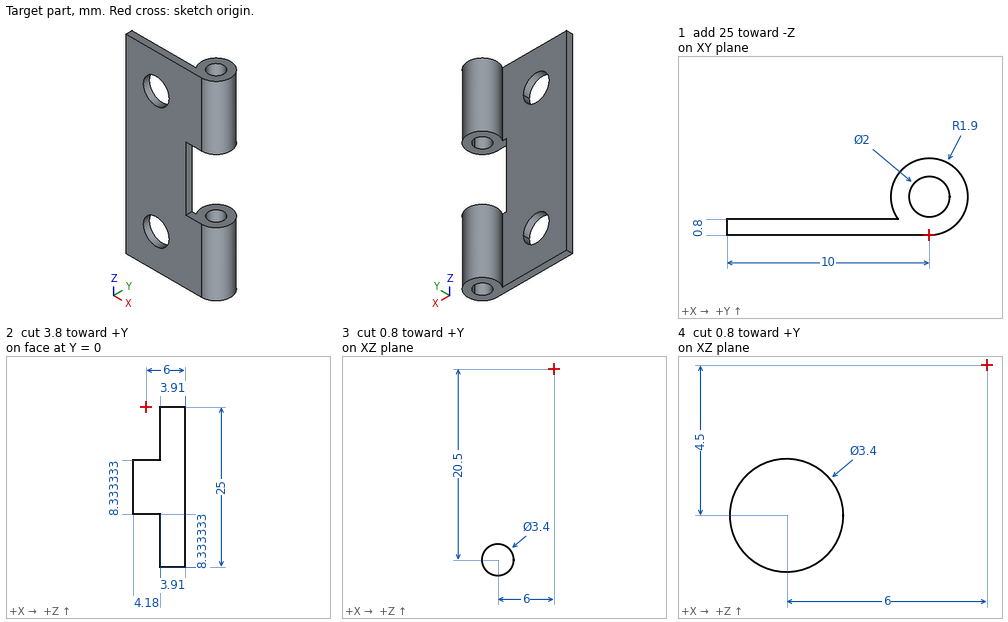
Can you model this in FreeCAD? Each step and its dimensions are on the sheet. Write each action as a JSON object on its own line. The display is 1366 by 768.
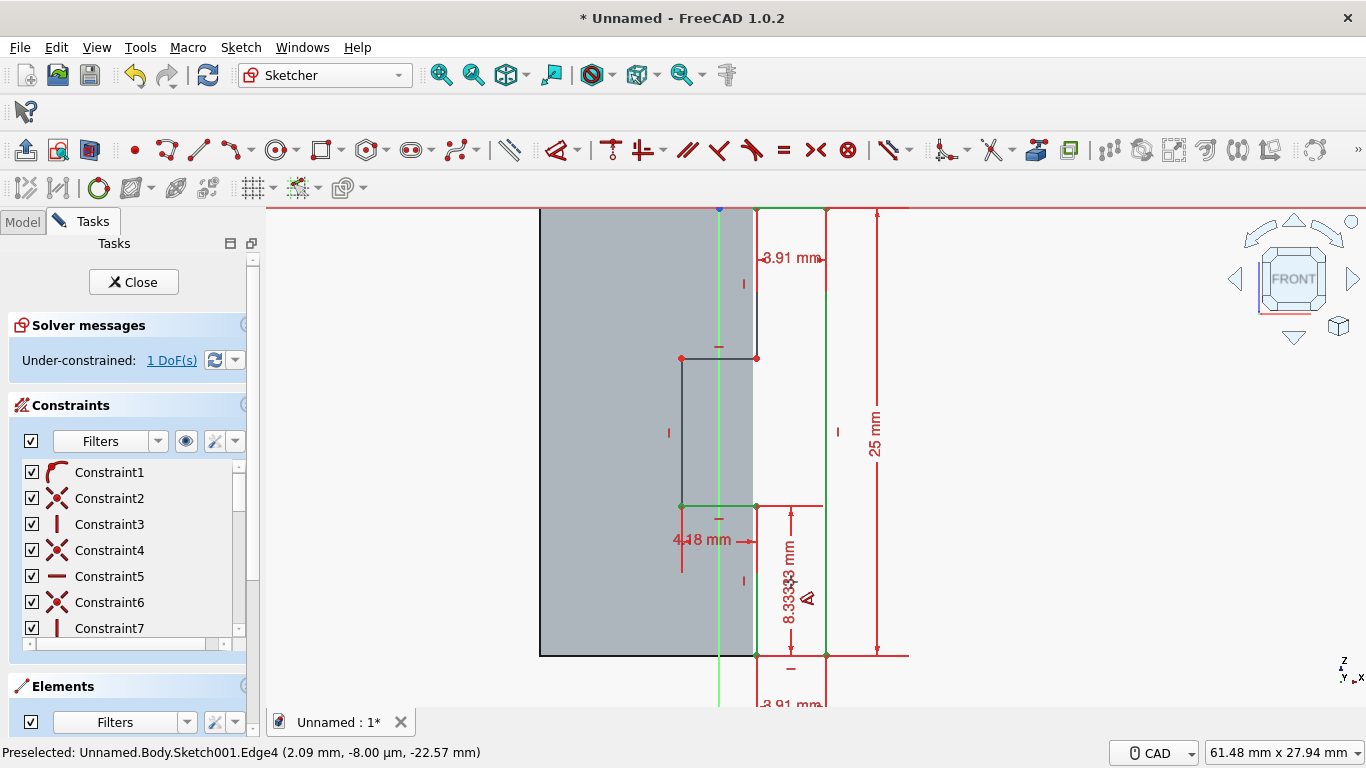
{"action": "left_click", "coordinate": [682, 462]}
{"action": "left_click", "coordinate": [648, 432]}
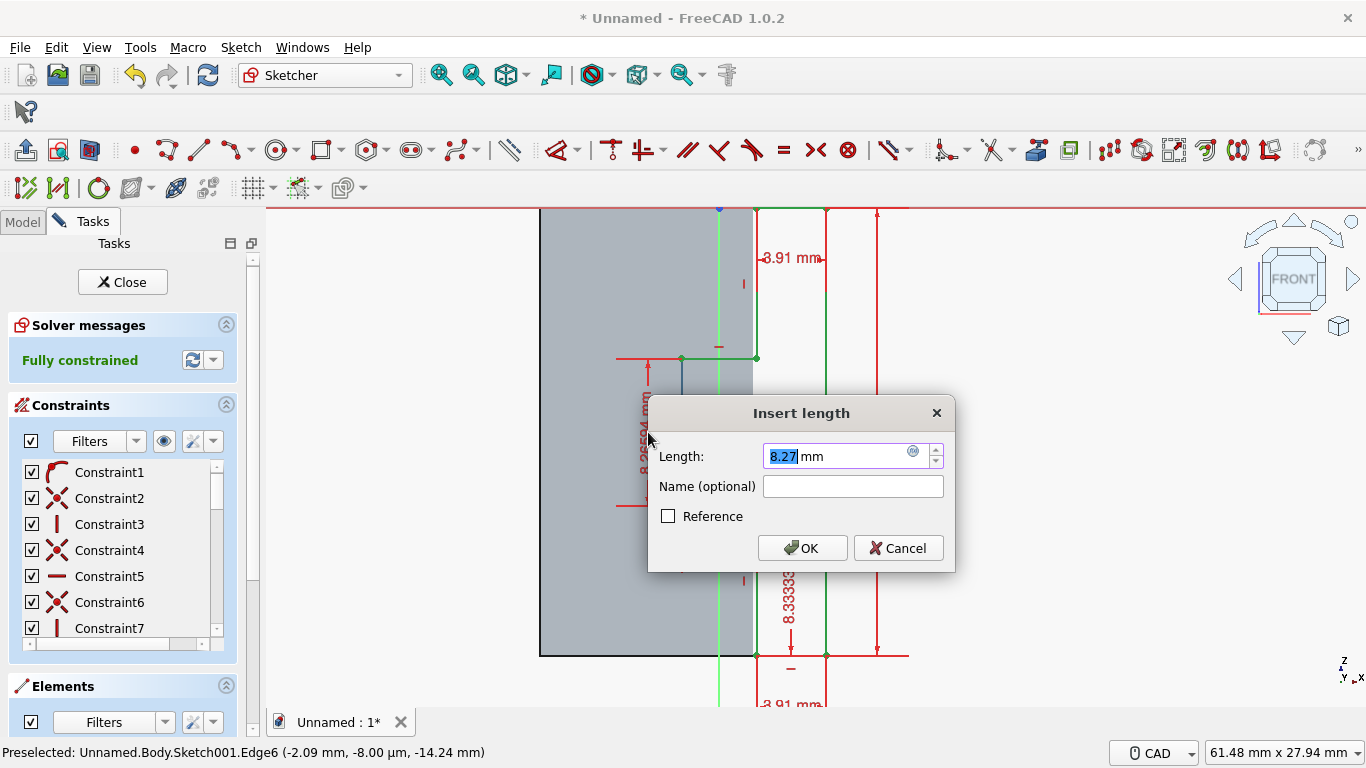
{"action": "type", "text": "8.333333"}
{"action": "key", "text": "Return"}
{"action": "key", "text": "Escape"}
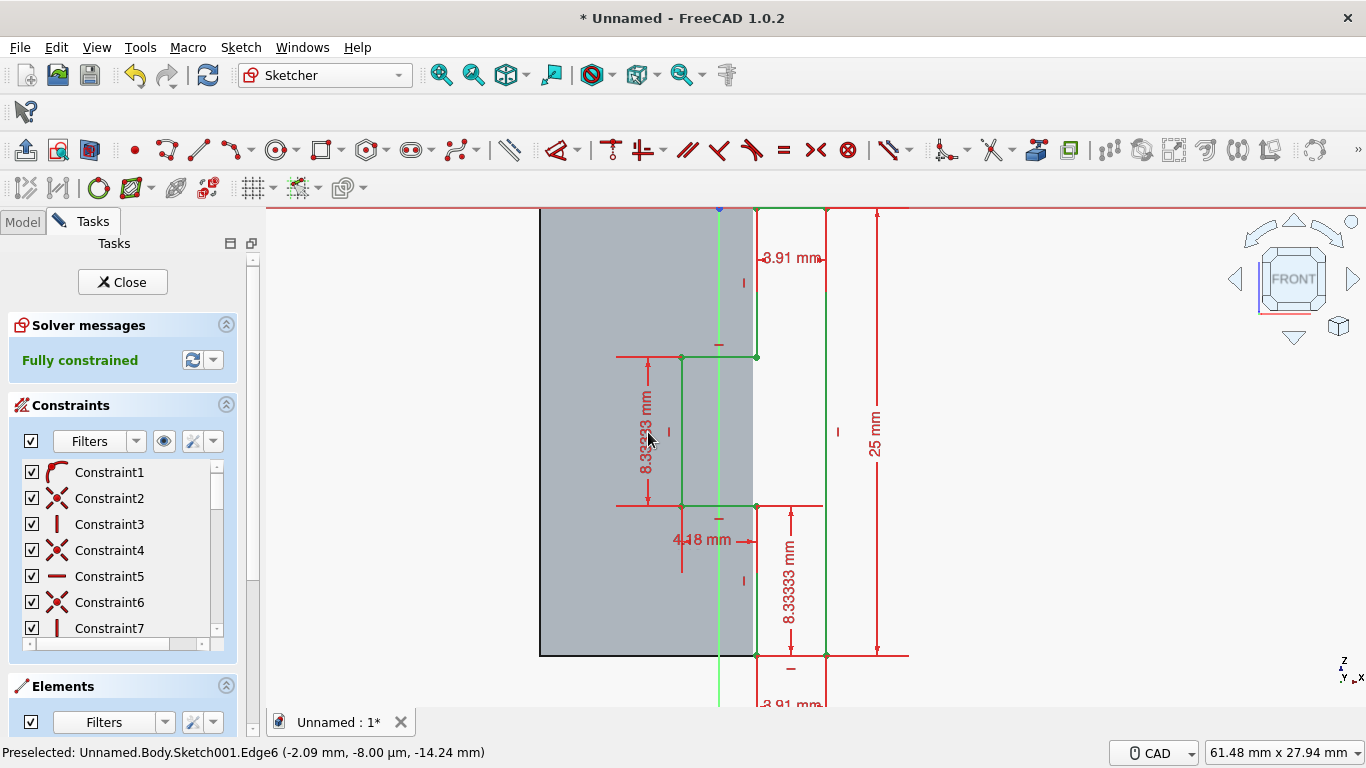
{"action": "left_click", "coordinate": [123, 282]}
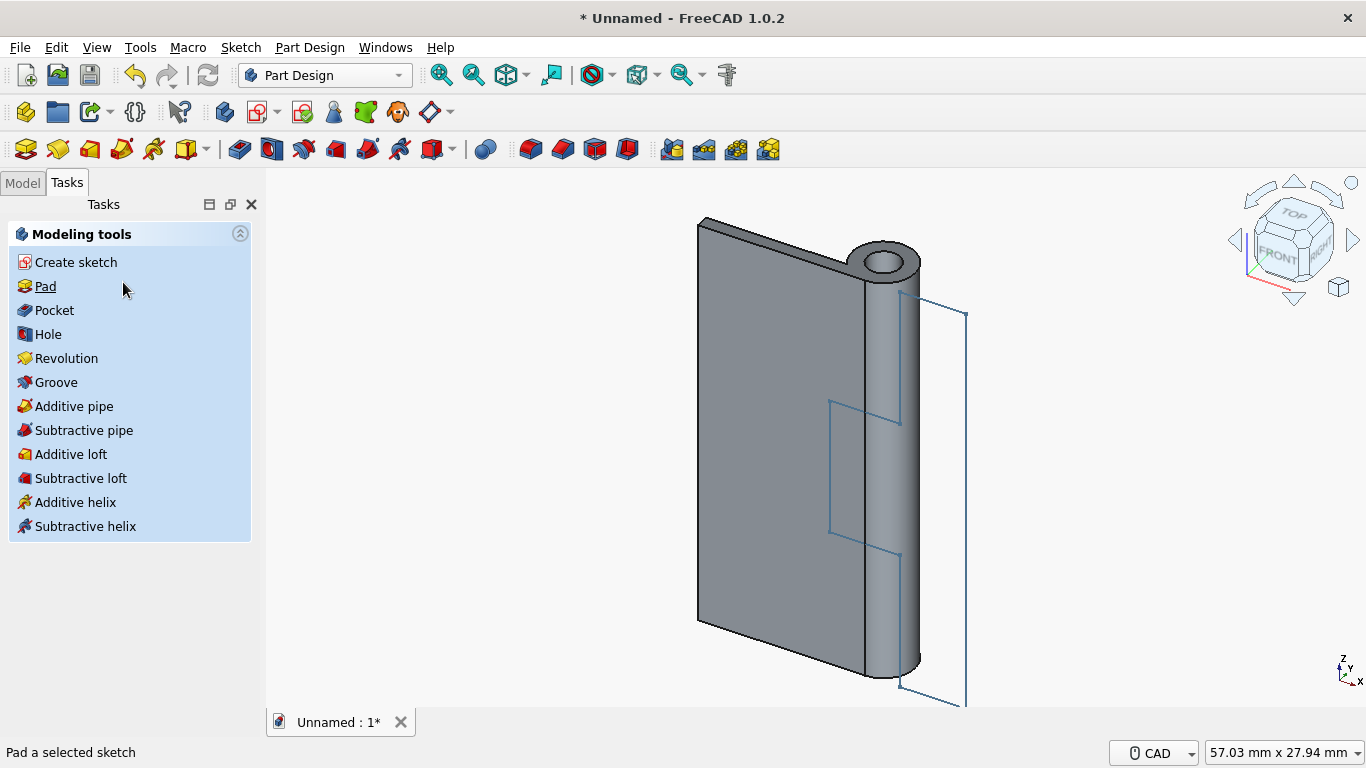
{"action": "left_click", "coordinate": [240, 150]}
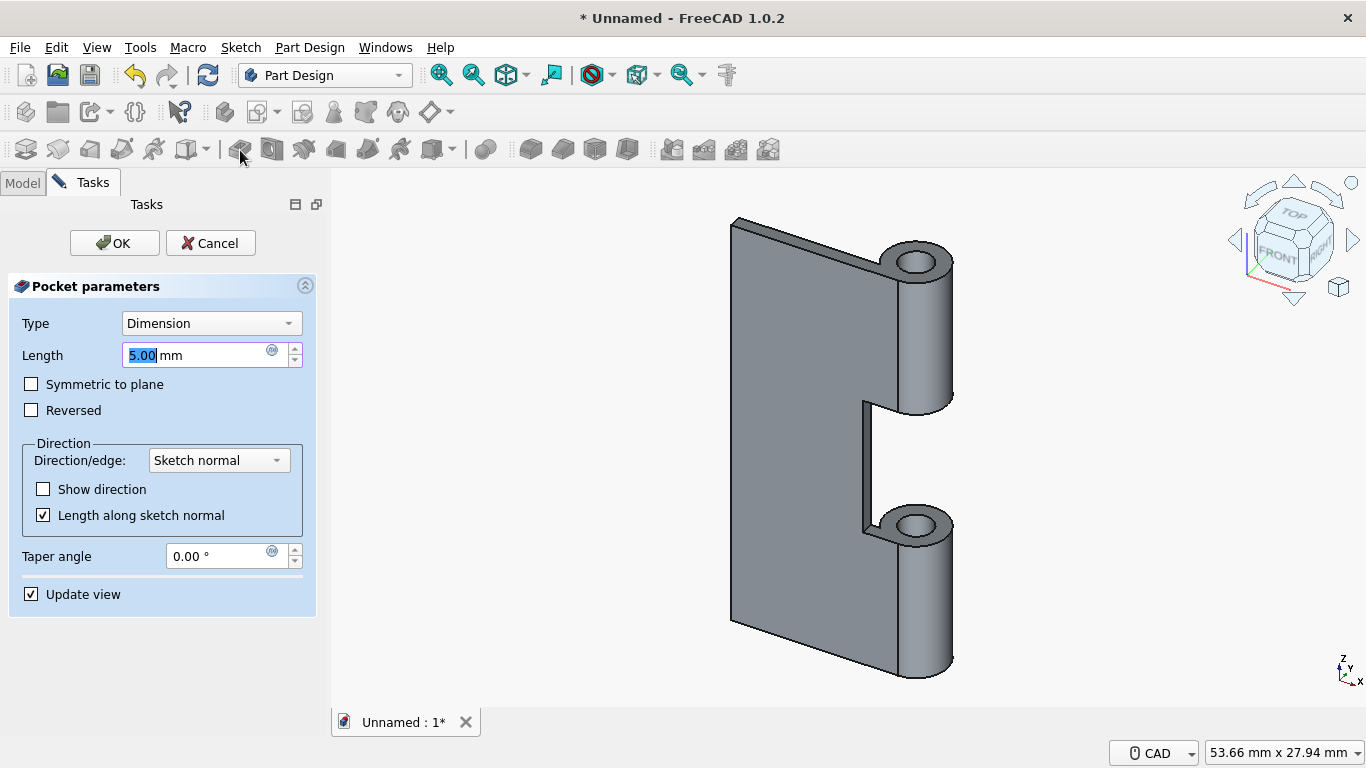
{"action": "type", "text": "3.8"}
{"action": "key", "text": "Tab"}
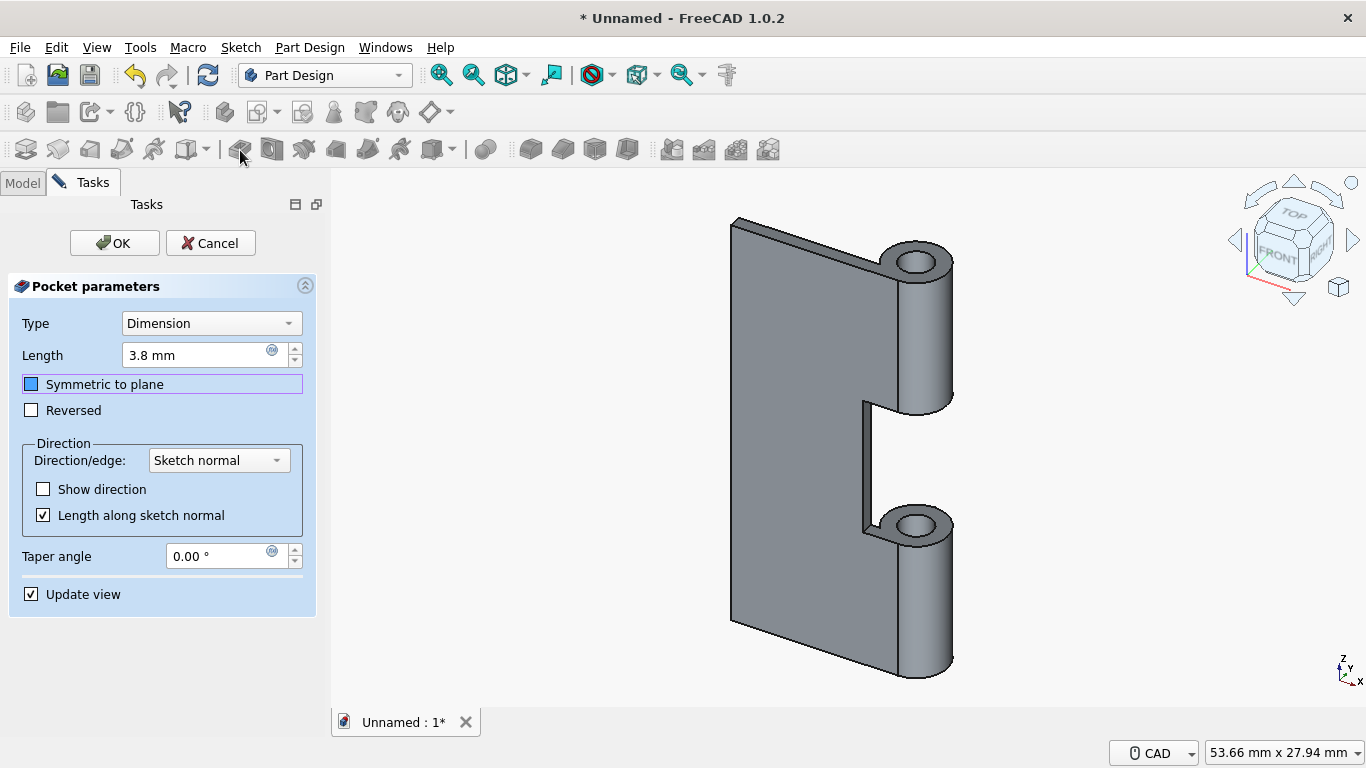
{"action": "left_click", "coordinate": [115, 243]}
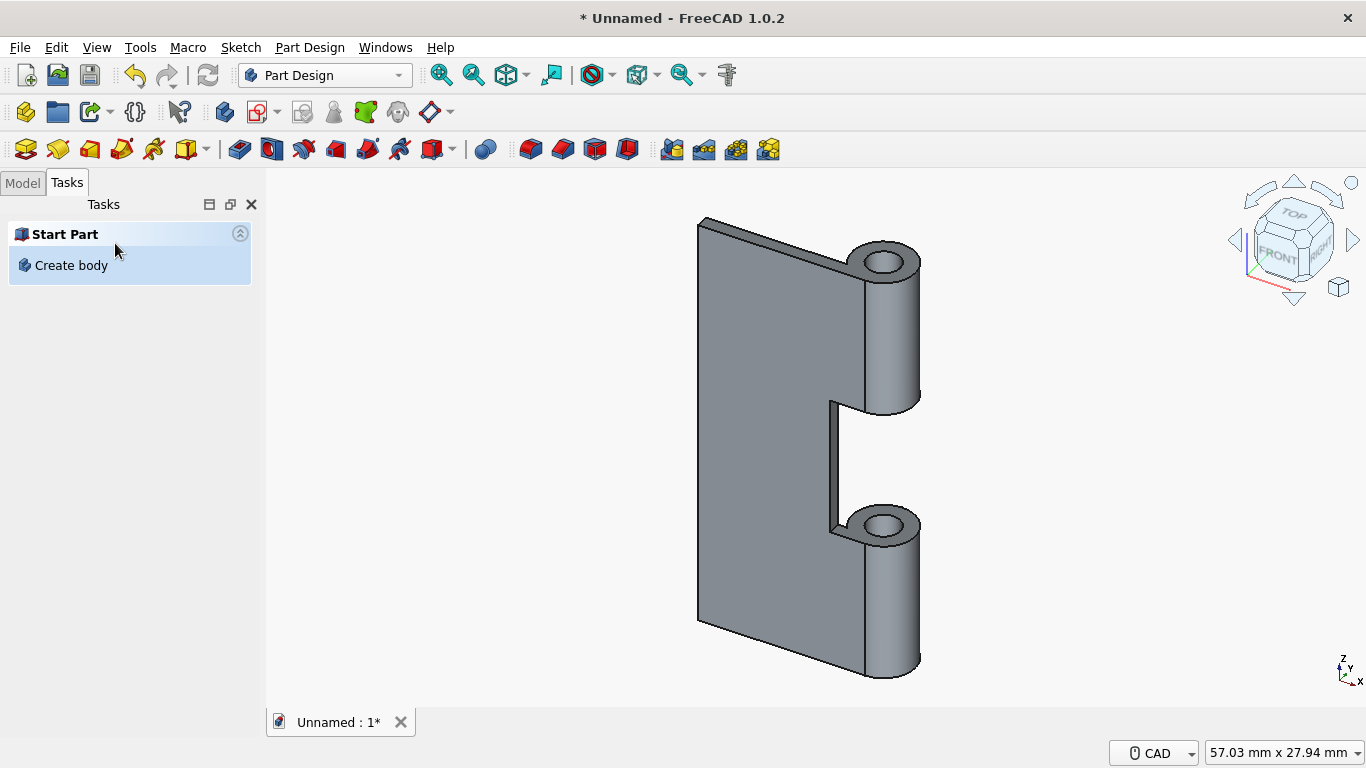
{"action": "left_click", "coordinate": [258, 112]}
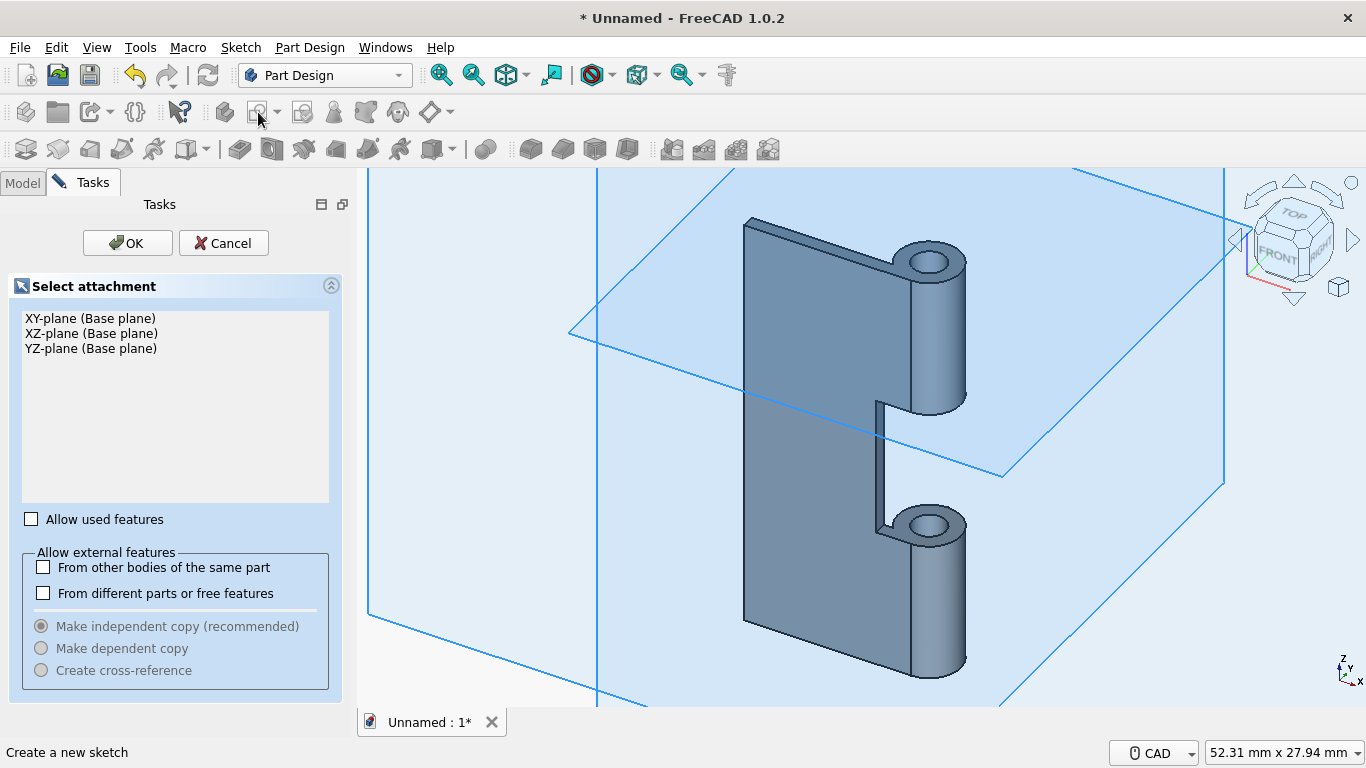
{"action": "left_click", "coordinate": [82, 334]}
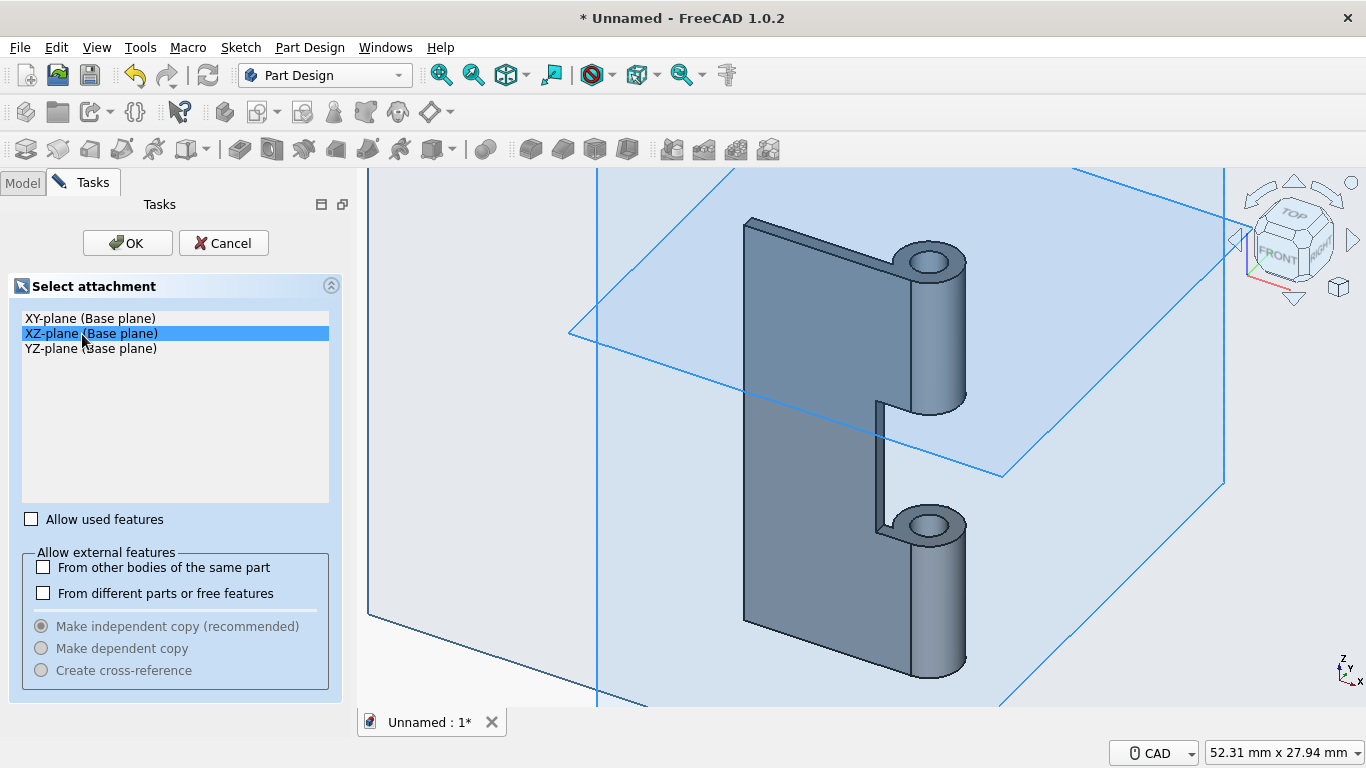
{"action": "left_click", "coordinate": [128, 243]}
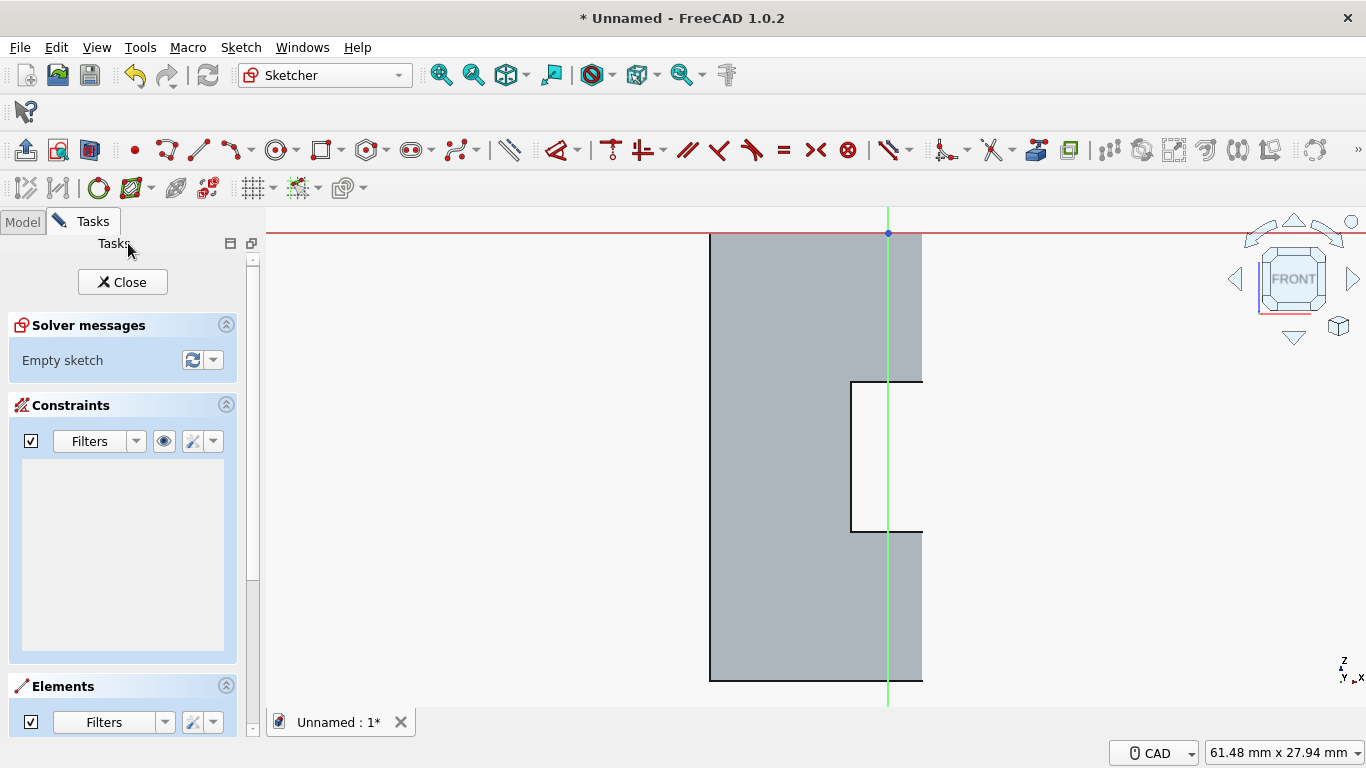
{"action": "scroll", "coordinate": [790, 636], "scroll_direction": "up", "scroll_amount": 8}